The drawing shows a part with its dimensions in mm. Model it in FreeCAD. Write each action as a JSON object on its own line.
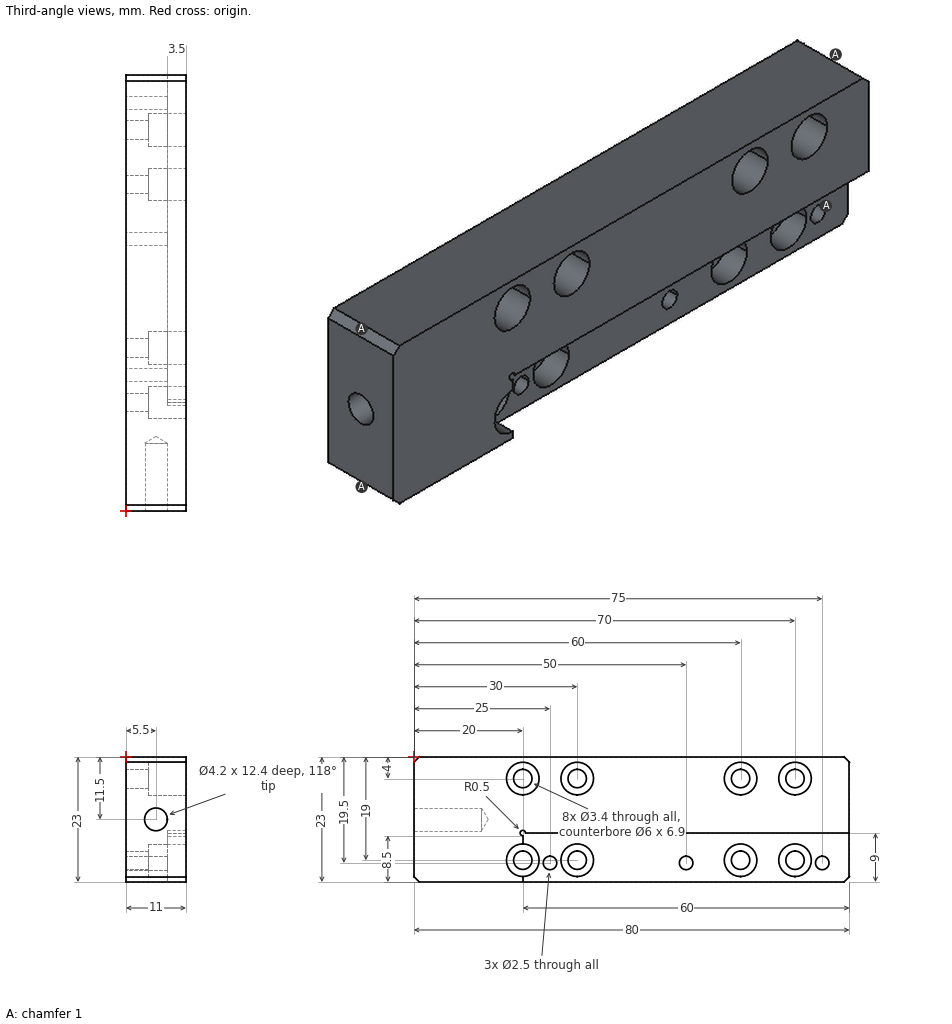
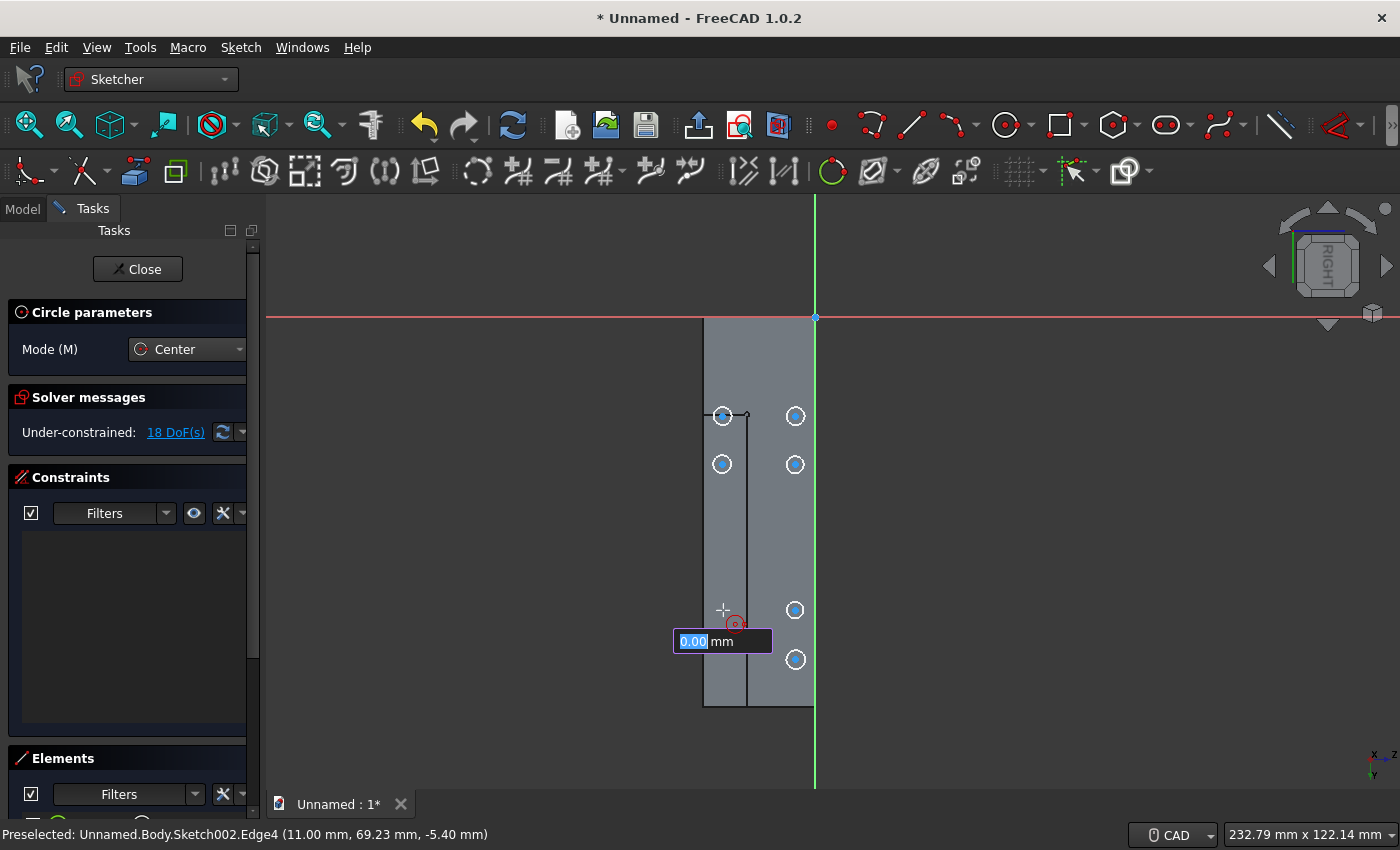
{"action": "scroll", "coordinate": [728, 604], "scroll_direction": "up", "scroll_amount": 4}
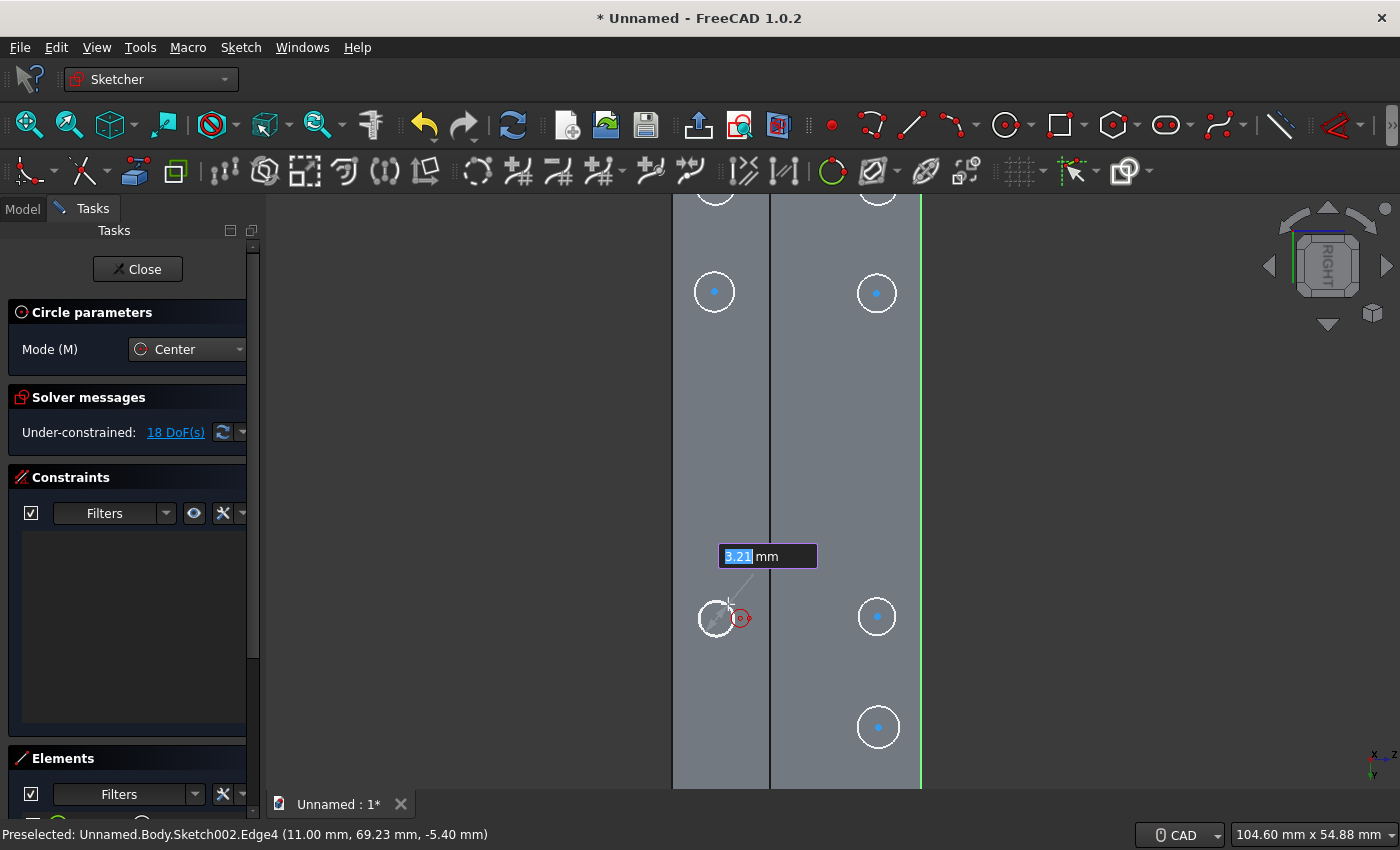
{"action": "left_click", "coordinate": [728, 603]}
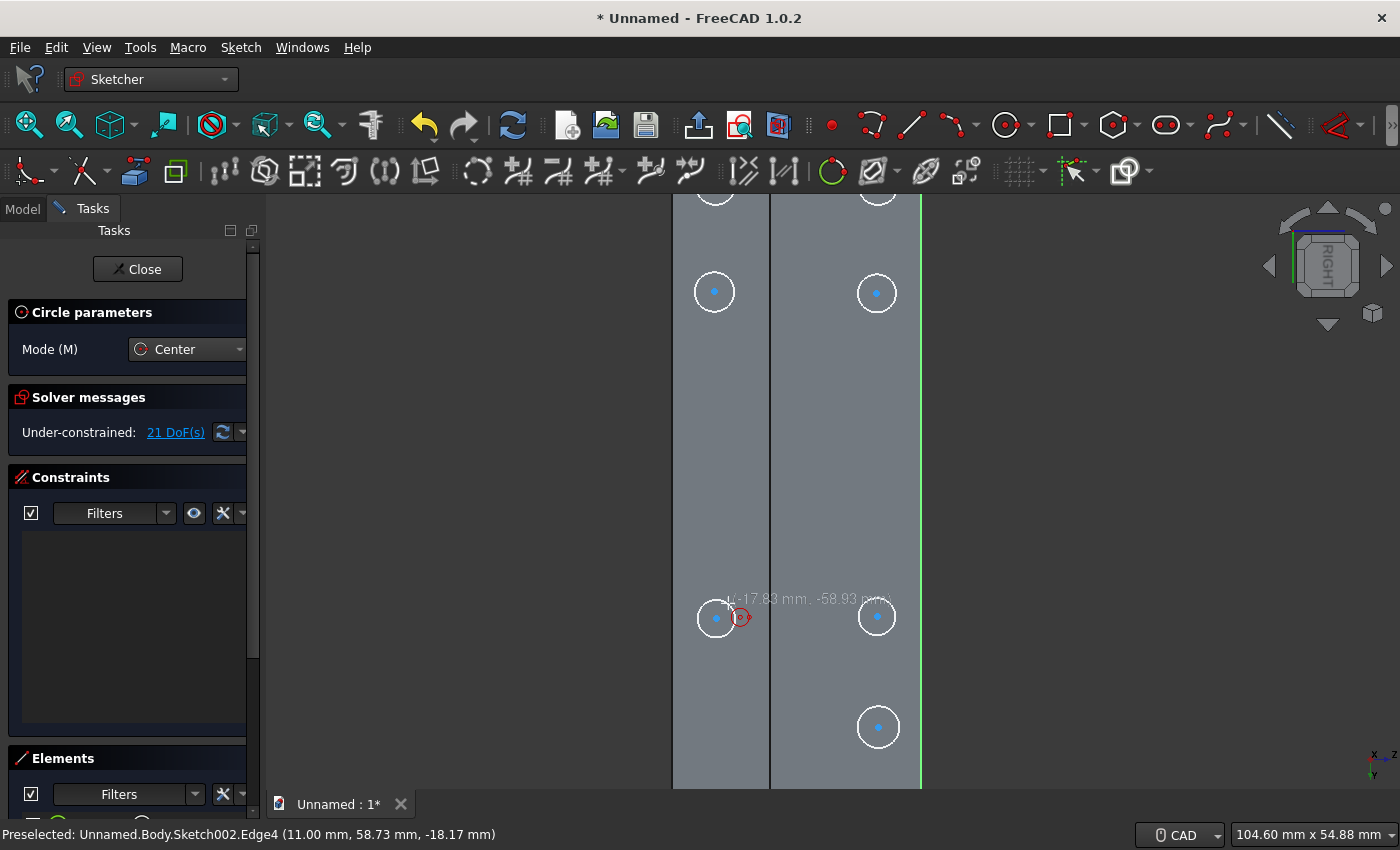
{"action": "scroll", "coordinate": [715, 724], "scroll_direction": "up", "scroll_amount": 2}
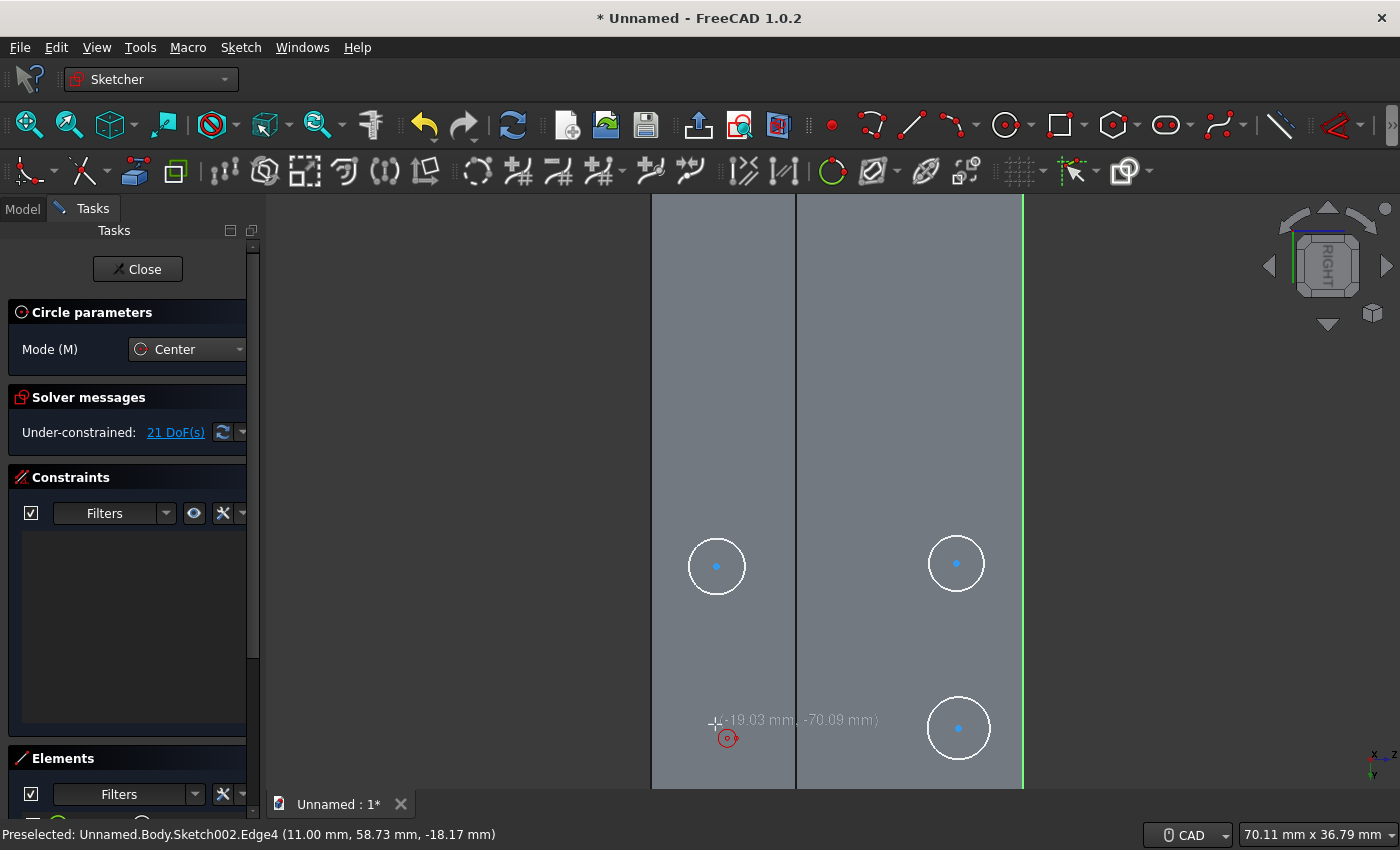
{"action": "scroll", "coordinate": [725, 630], "scroll_direction": "down", "scroll_amount": 6}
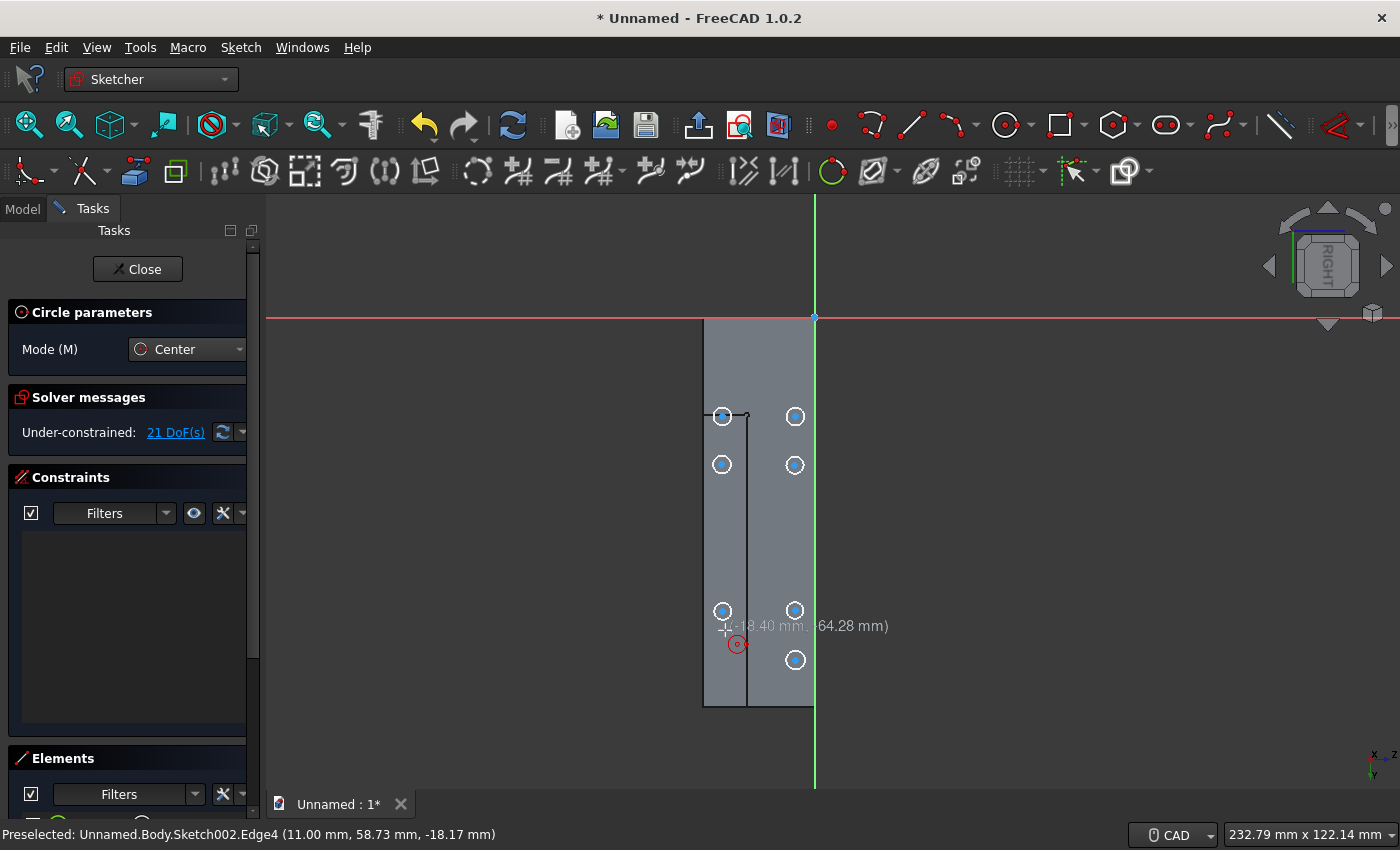
{"action": "left_click", "coordinate": [722, 659]}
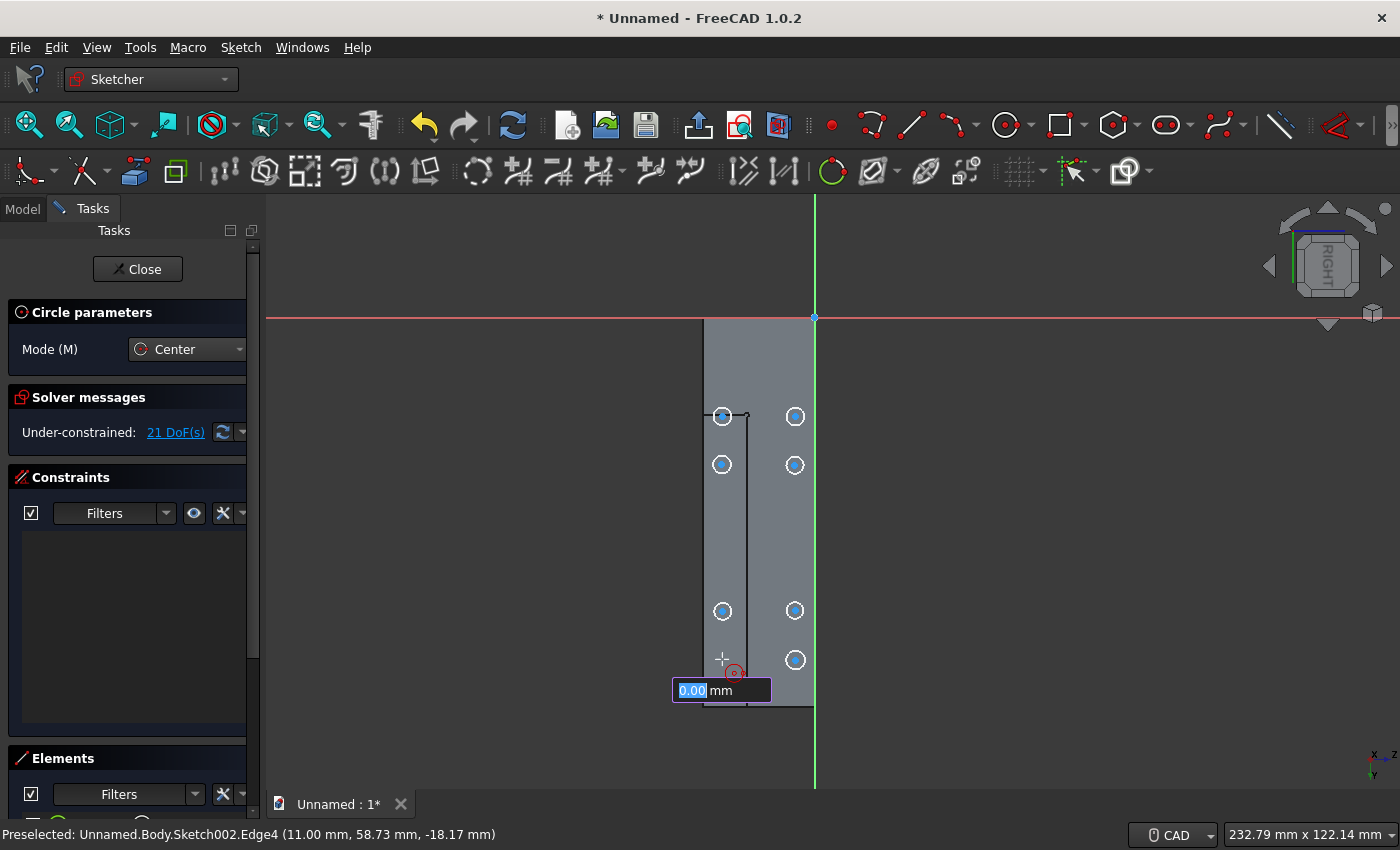
{"action": "scroll", "coordinate": [728, 653], "scroll_direction": "up", "scroll_amount": 4}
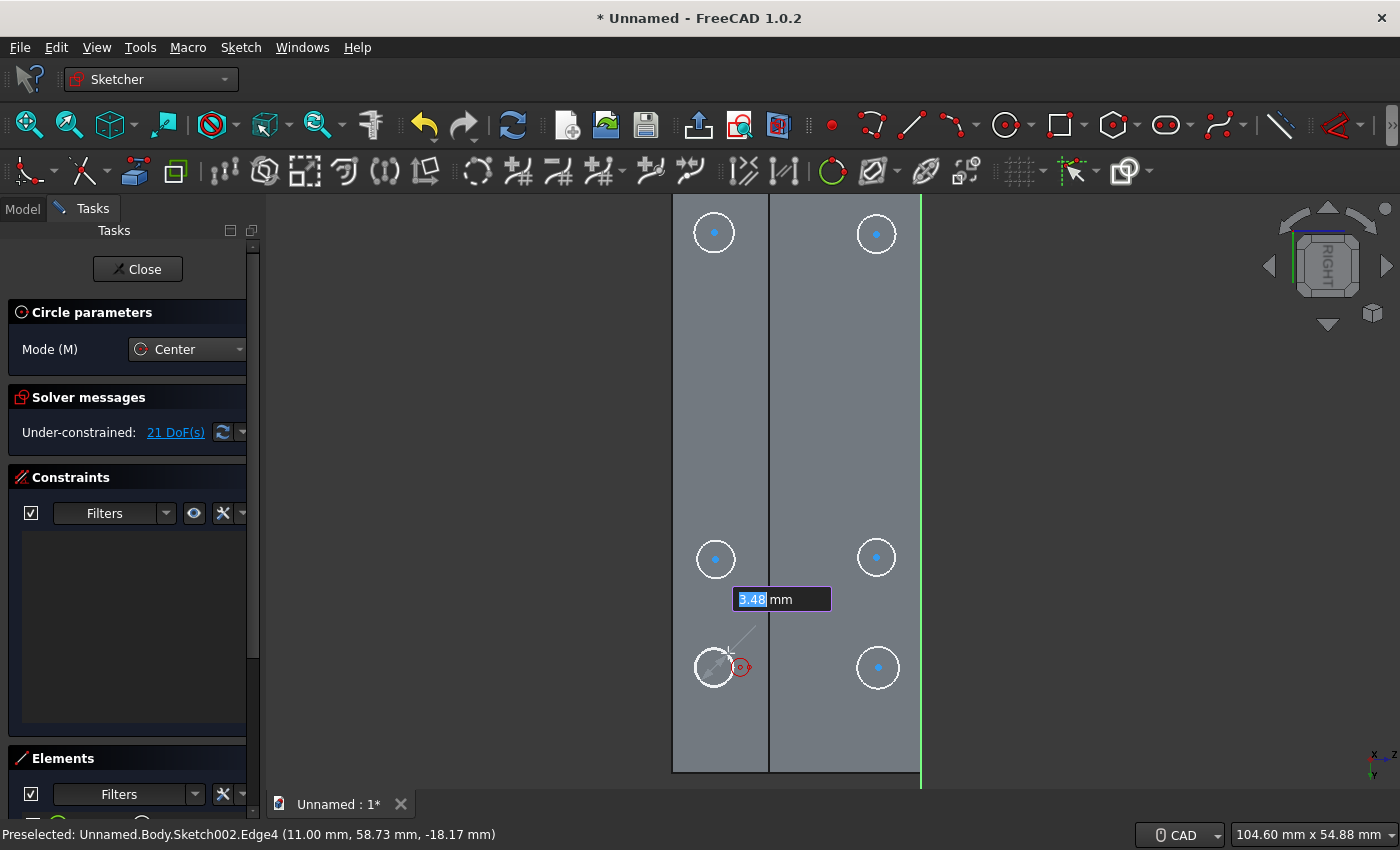
{"action": "left_click", "coordinate": [728, 652]}
{"action": "key", "text": "Escape"}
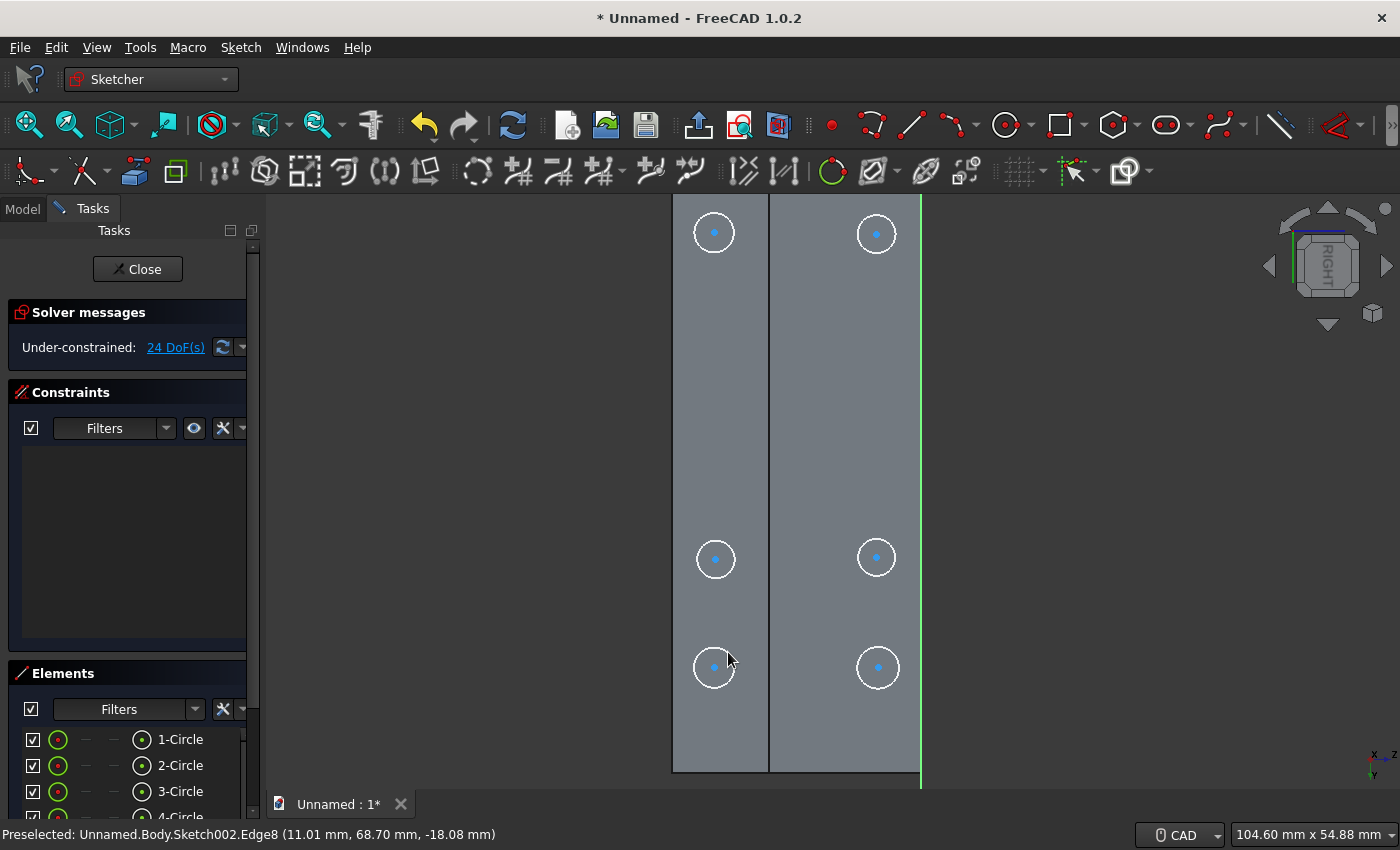
{"action": "scroll", "coordinate": [728, 652], "scroll_direction": "down", "scroll_amount": 4}